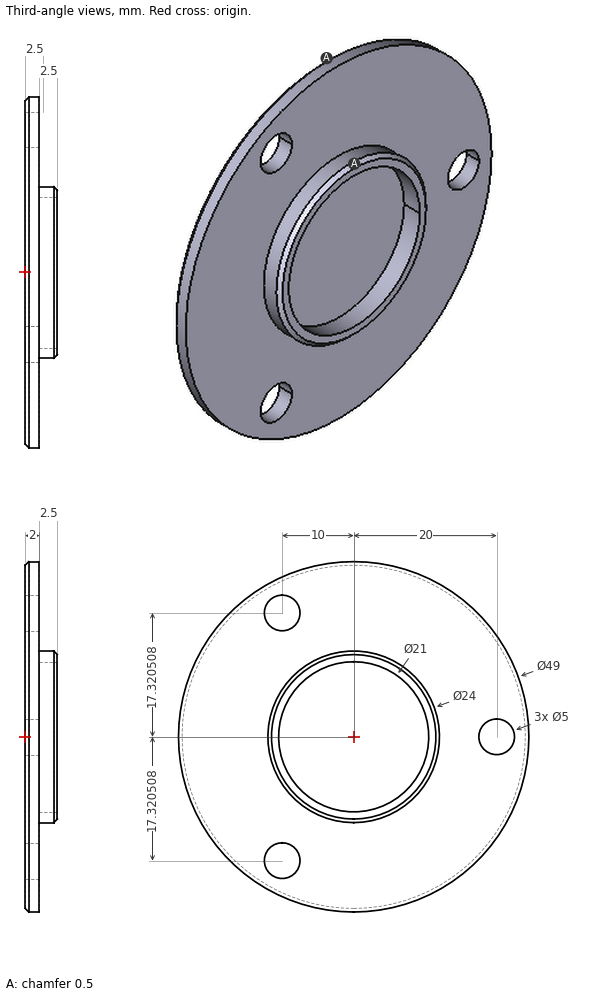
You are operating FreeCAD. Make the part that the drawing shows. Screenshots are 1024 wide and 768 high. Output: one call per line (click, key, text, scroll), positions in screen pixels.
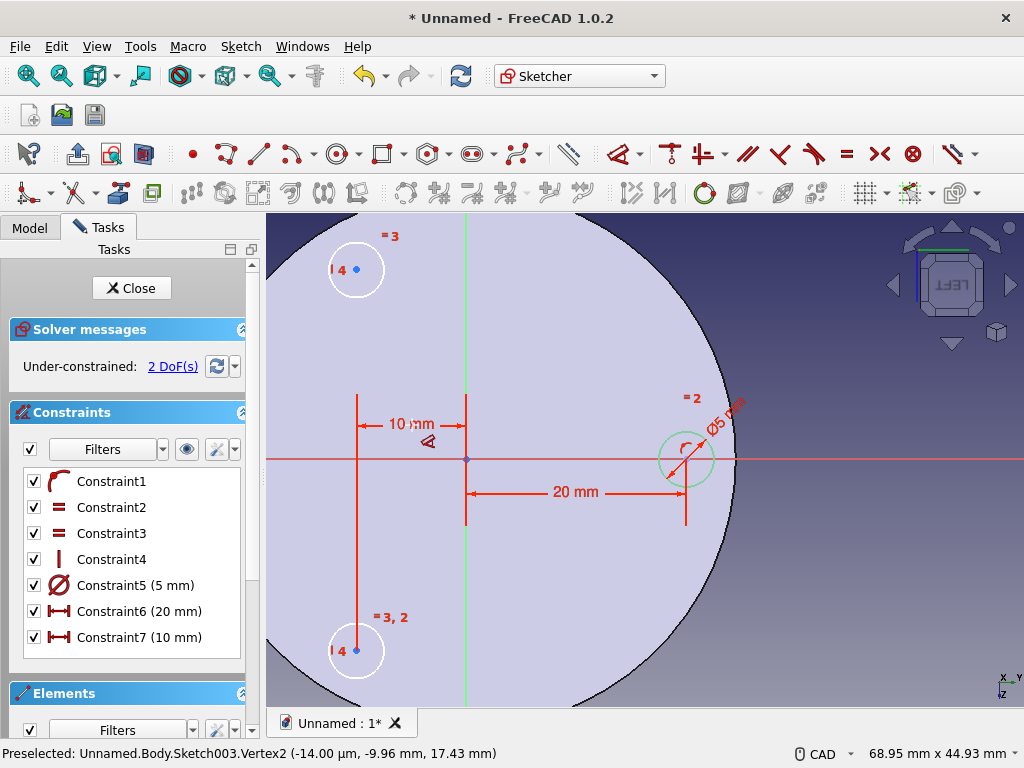
click(357, 651)
click(323, 555)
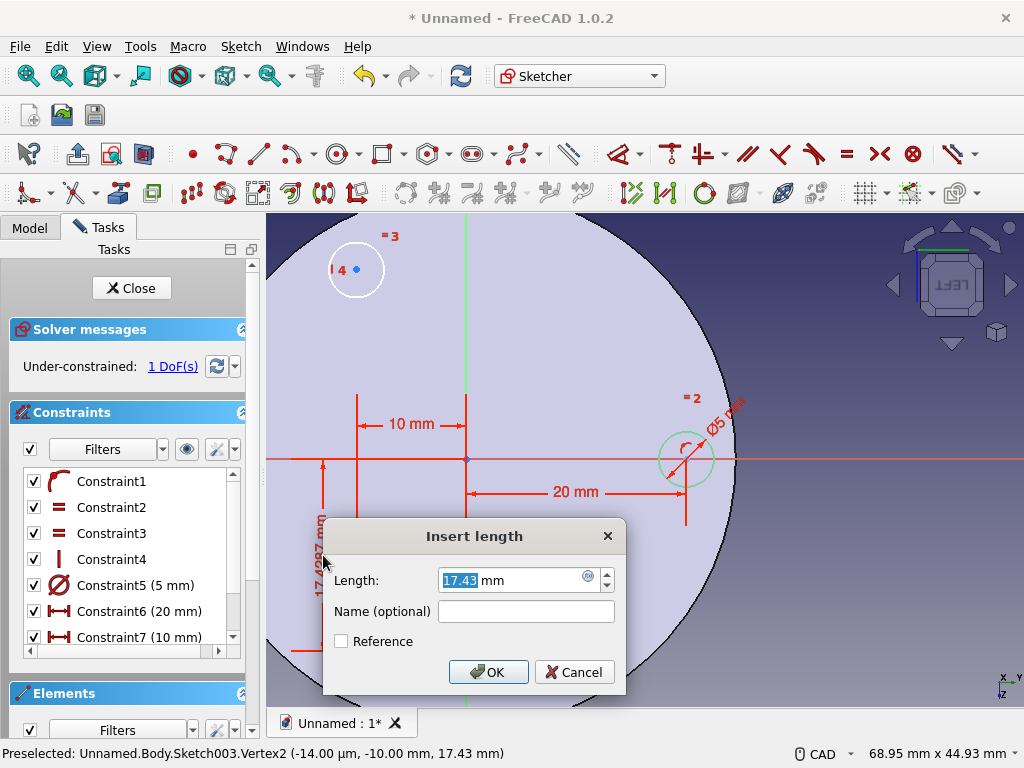
text(17.320508)
key(Return)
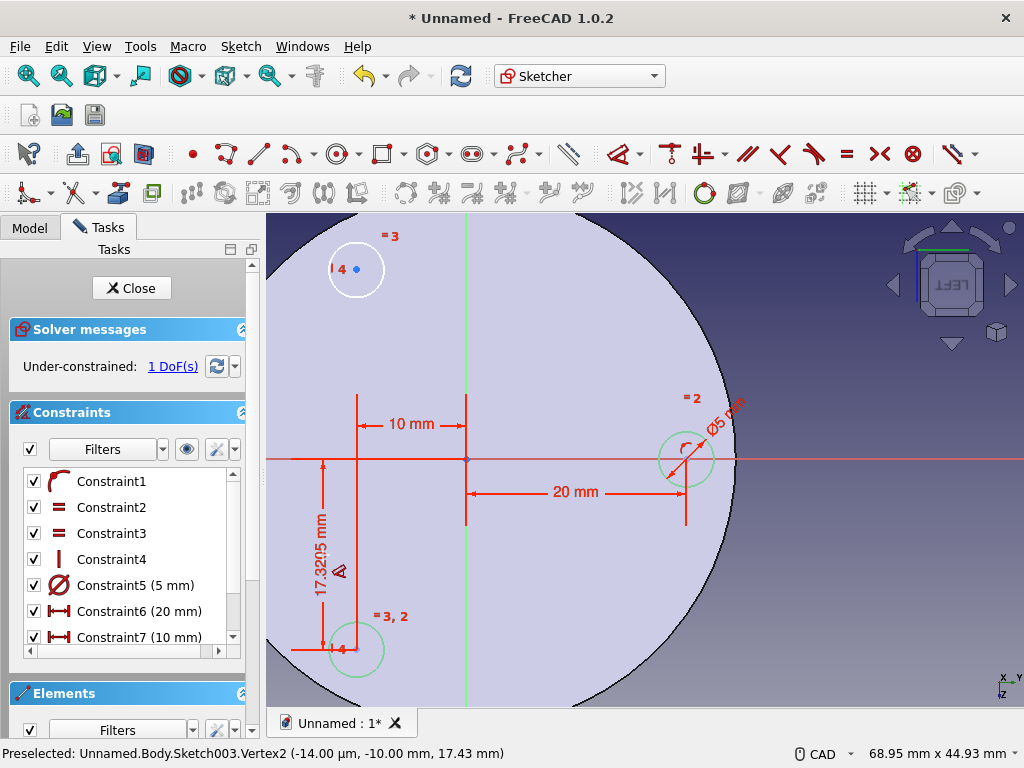
click(357, 270)
click(323, 365)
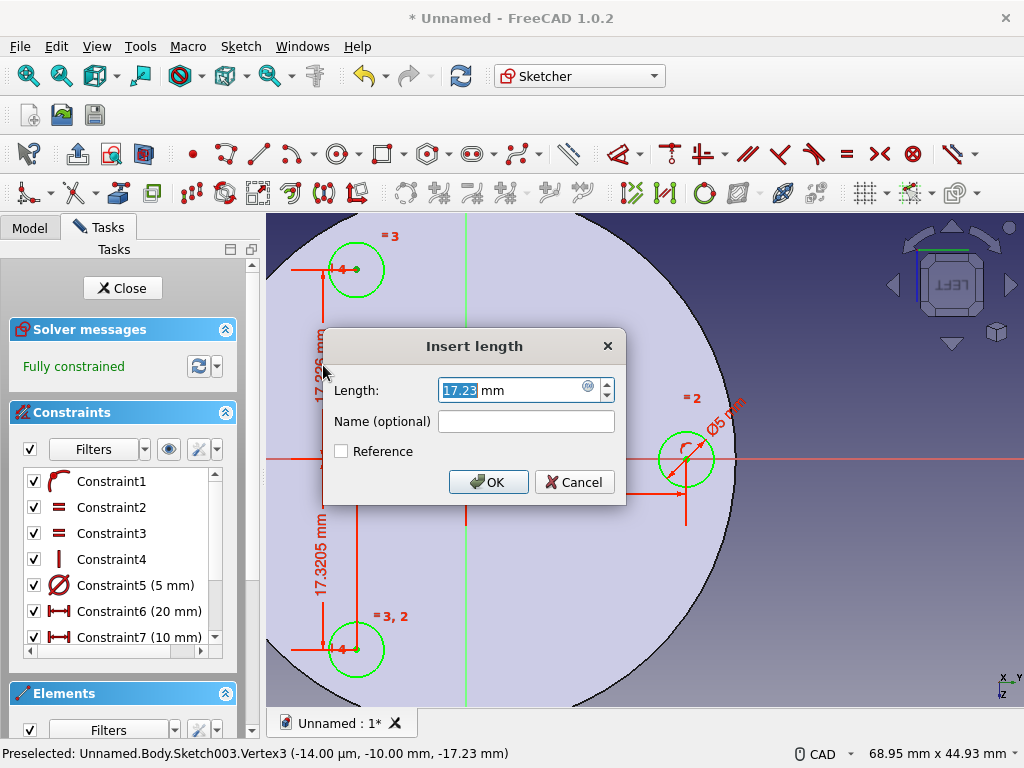
text(17.320508)
key(Return)
key(Escape)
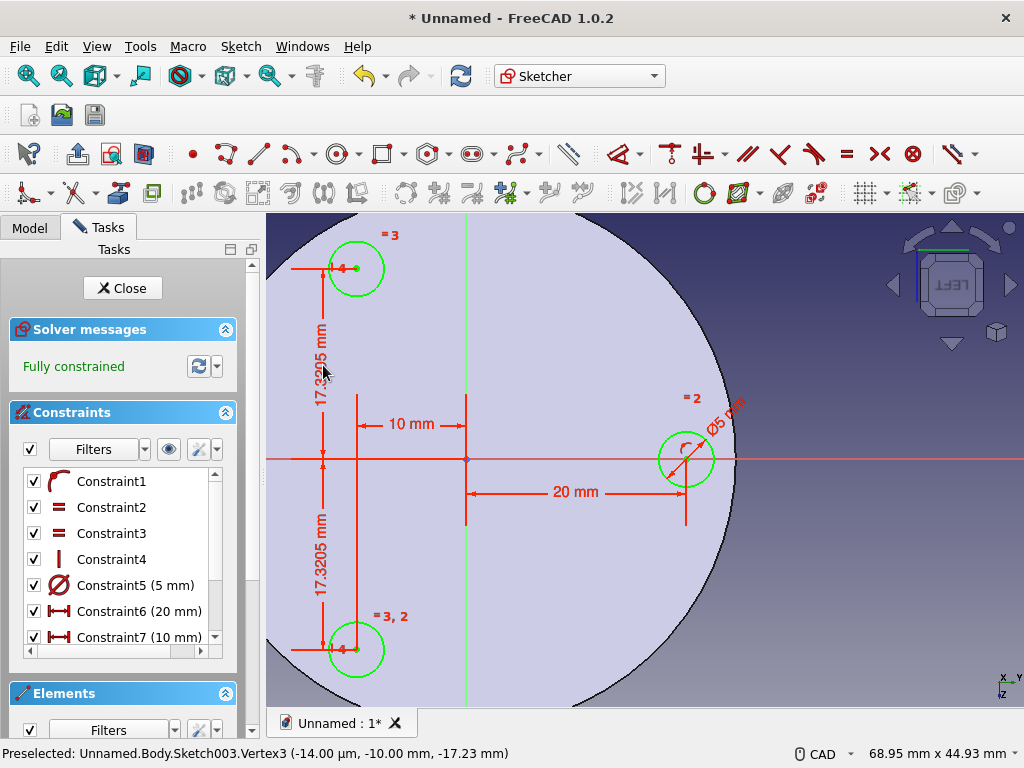
click(123, 288)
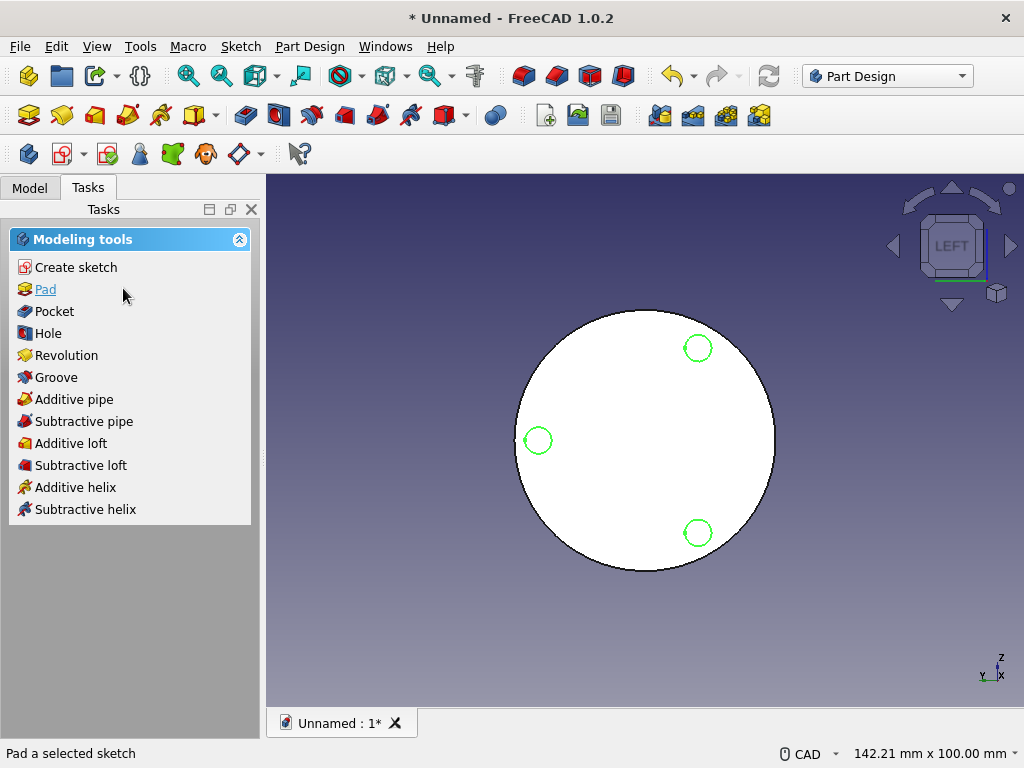
click(246, 116)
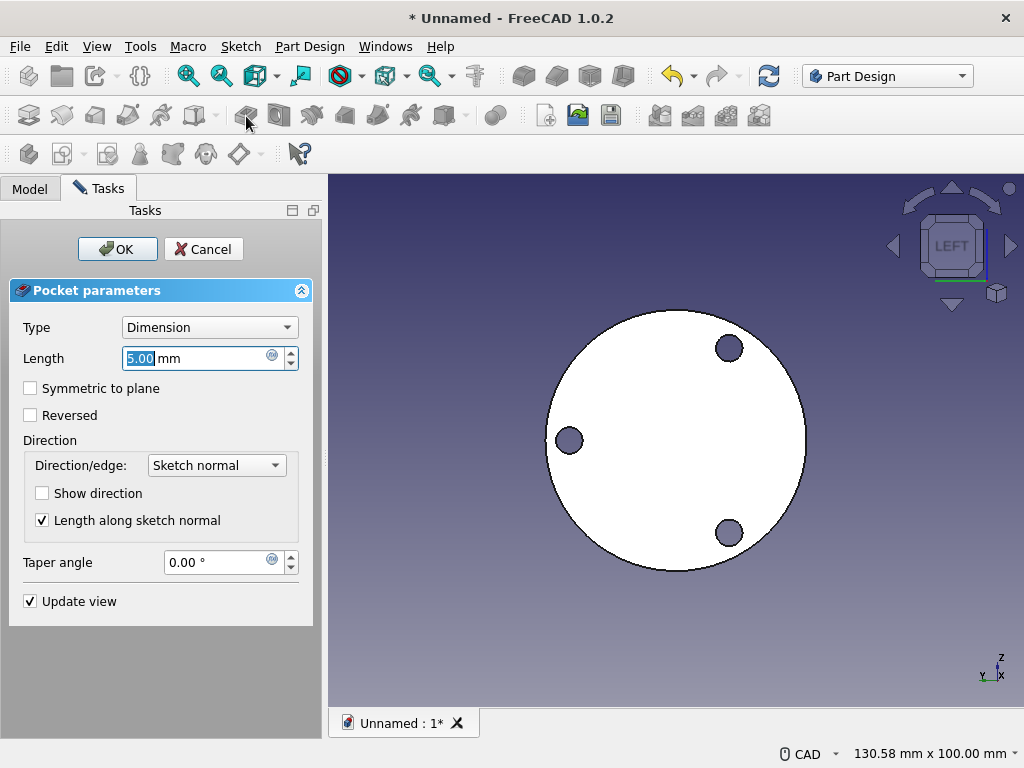
text(2.5)
key(Tab)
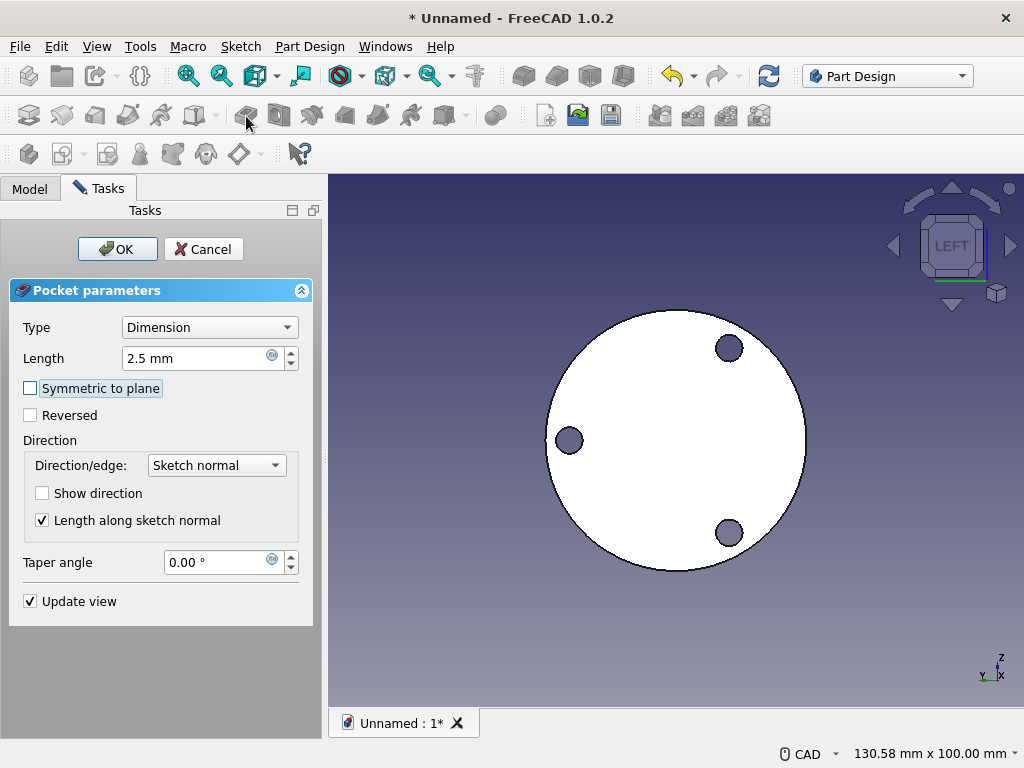
click(118, 249)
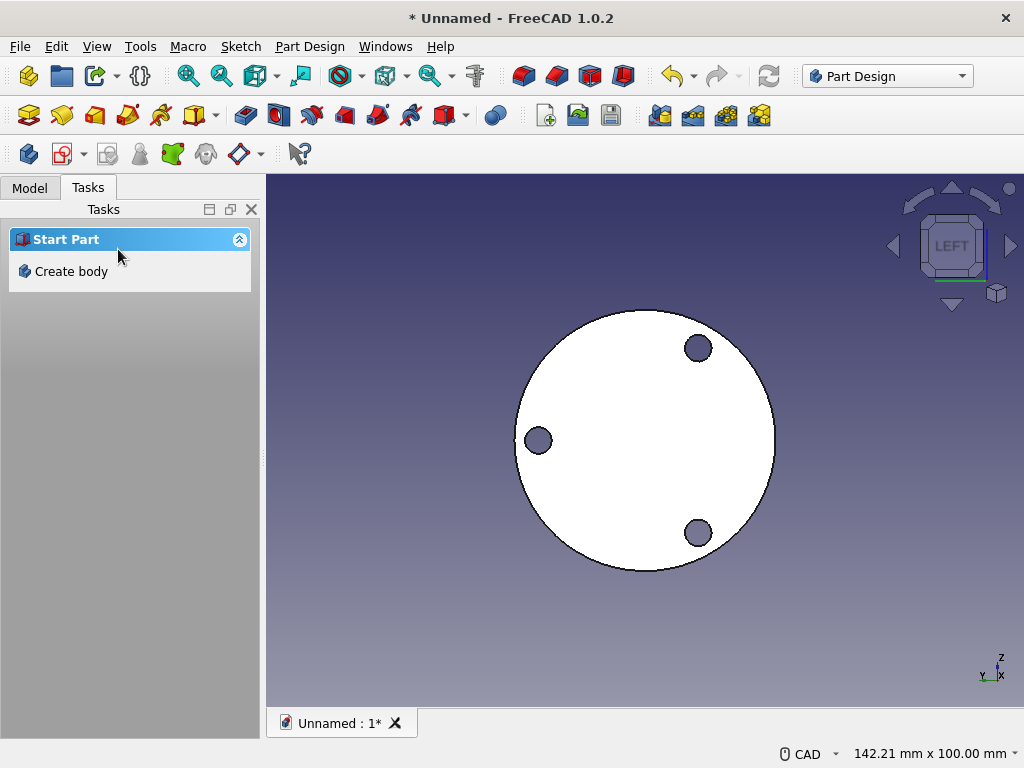
click(751, 363)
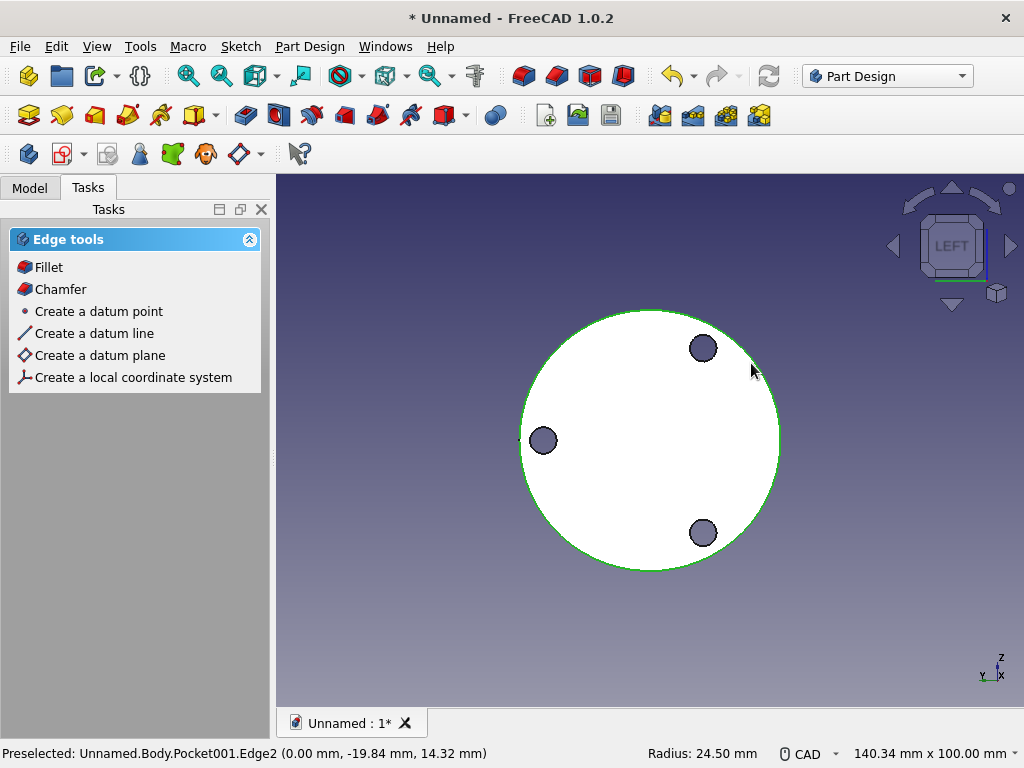
key(0)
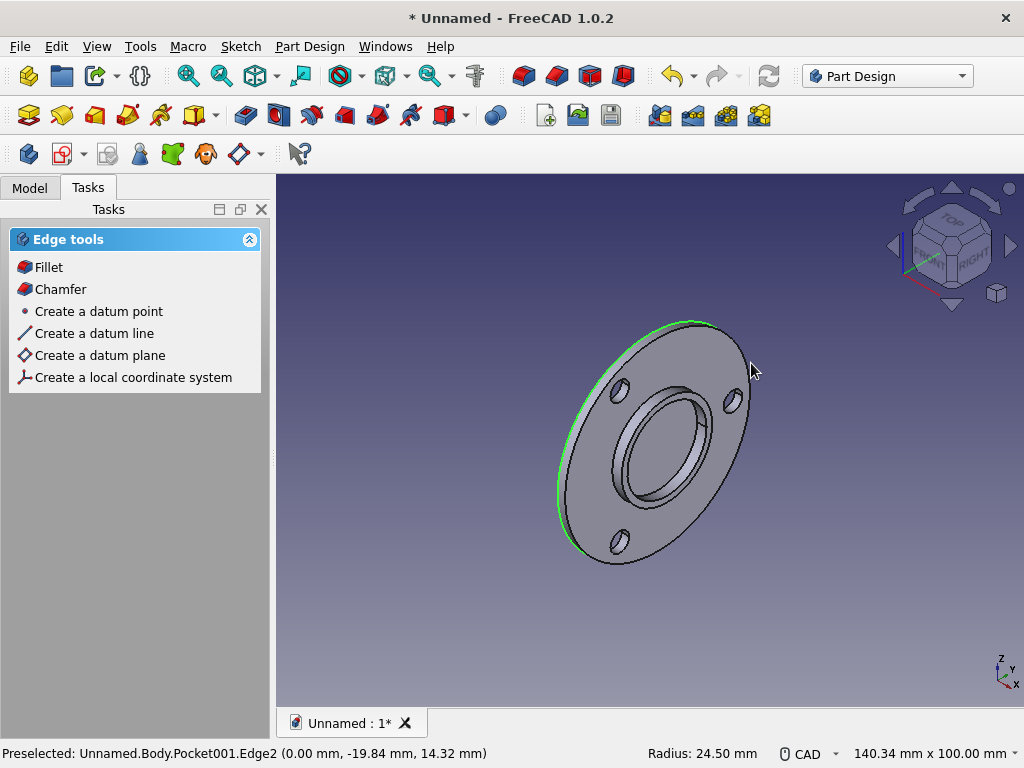
click(622, 475, ctrl)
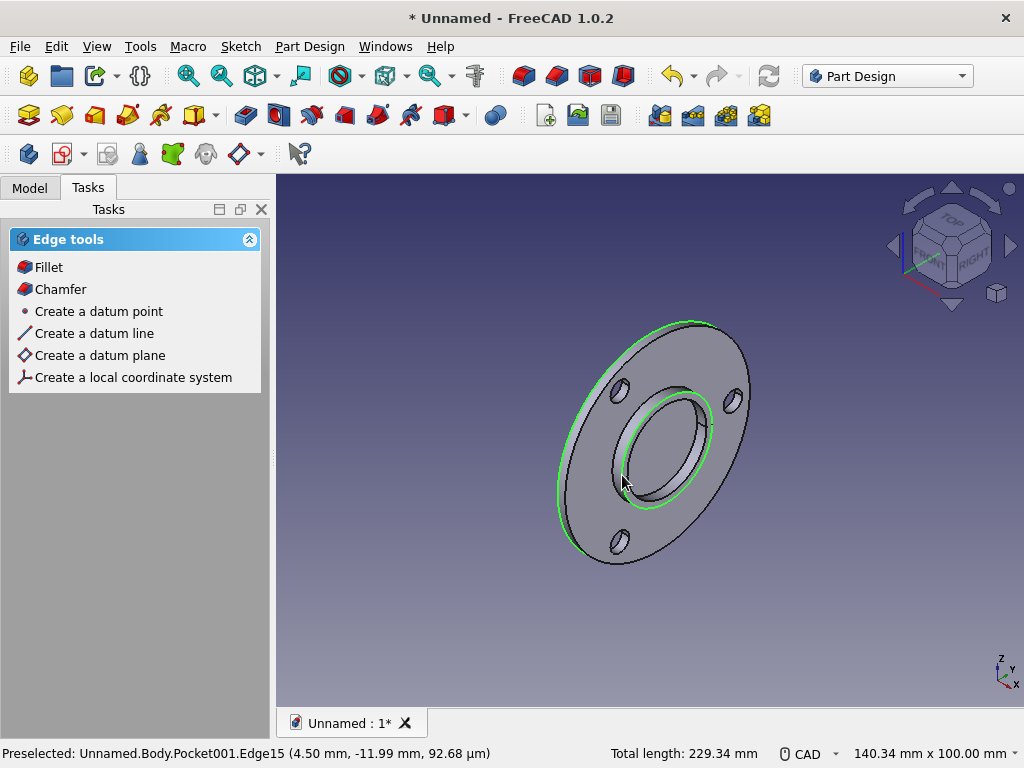
click(557, 76)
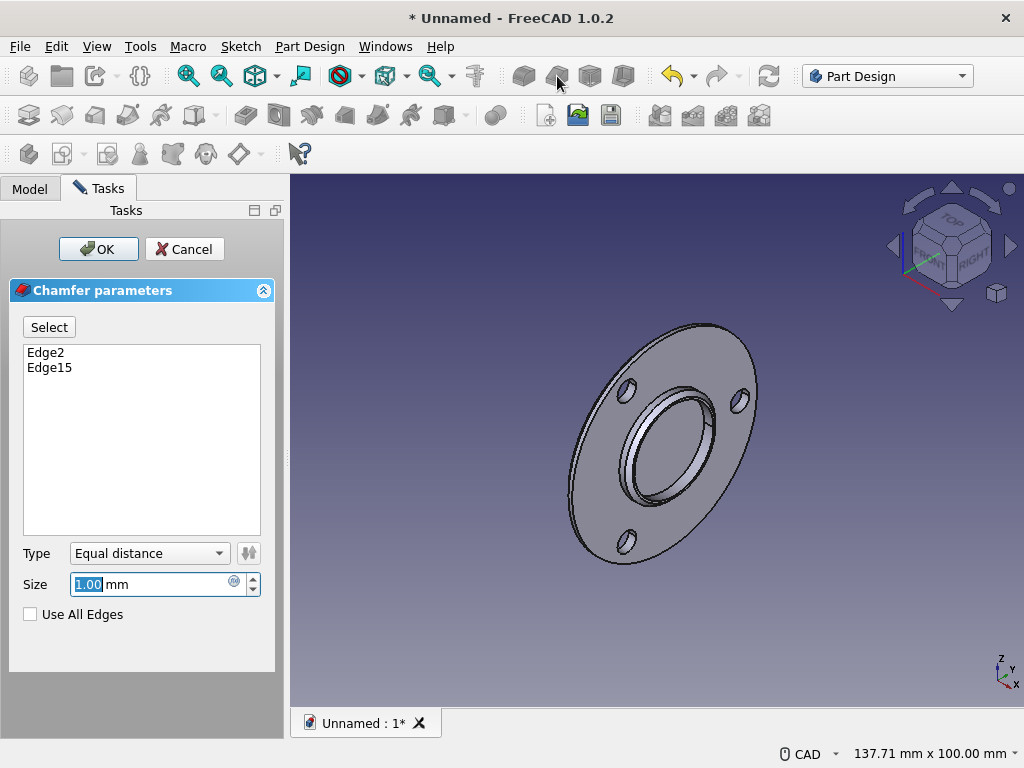
text(0.5)
key(Tab)